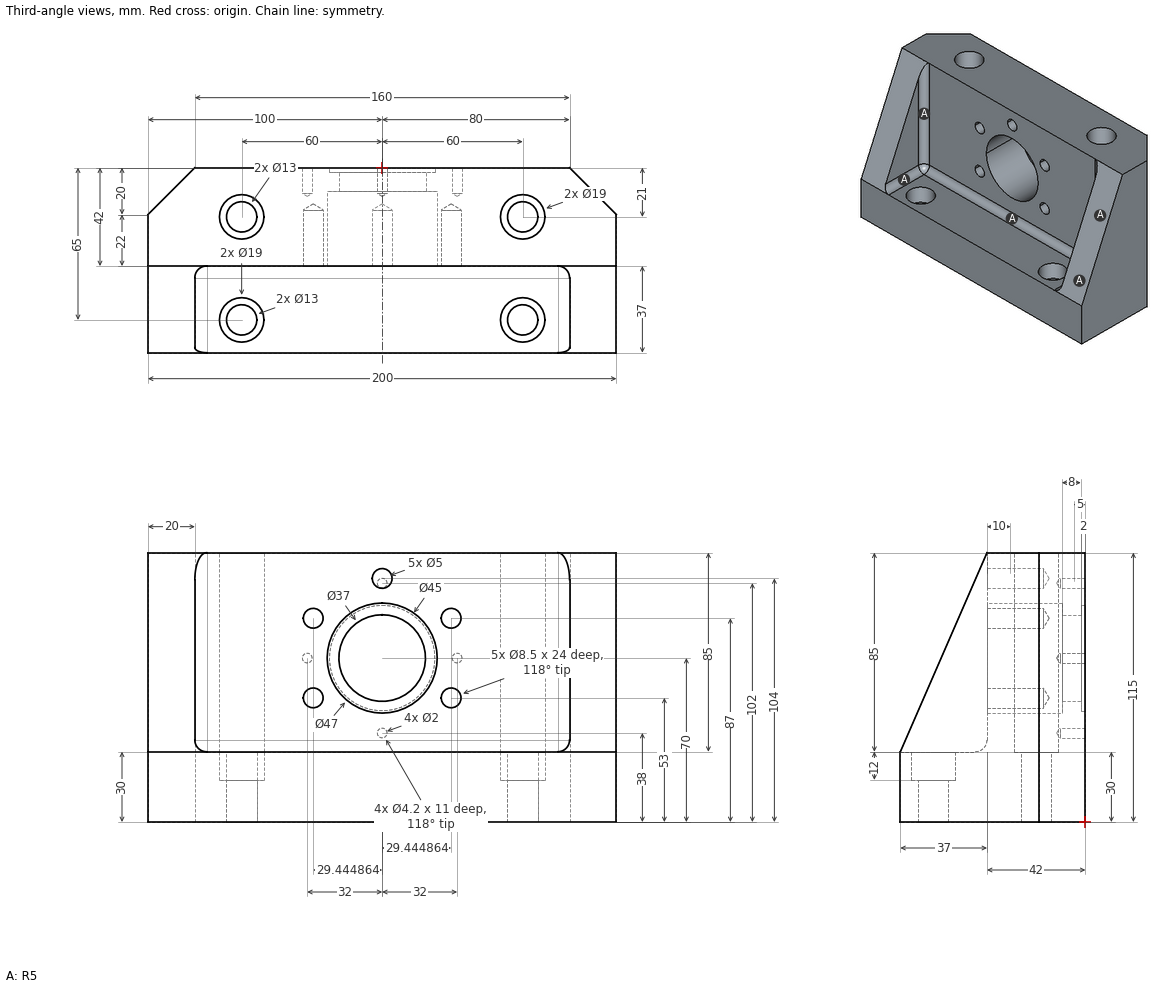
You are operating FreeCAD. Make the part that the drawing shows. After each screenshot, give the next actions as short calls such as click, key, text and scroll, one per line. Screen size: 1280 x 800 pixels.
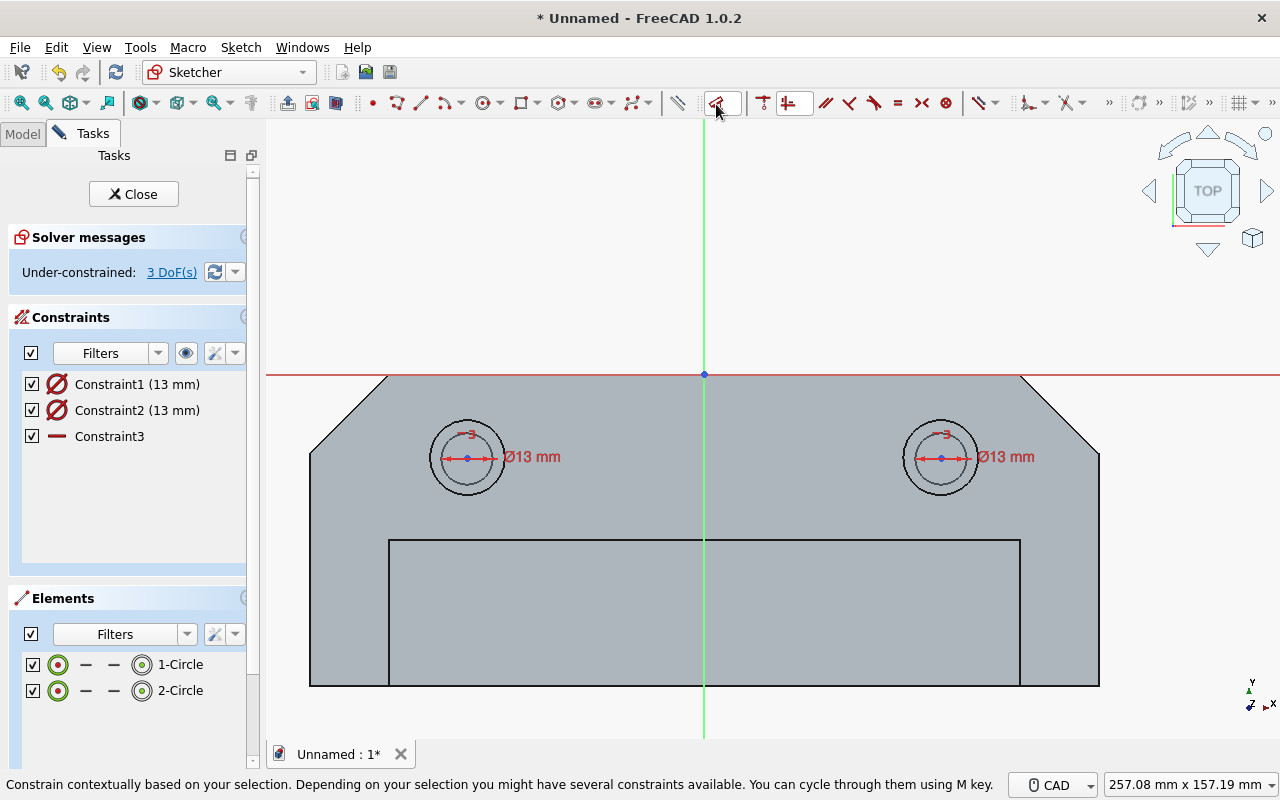
click(467, 459)
click(586, 341)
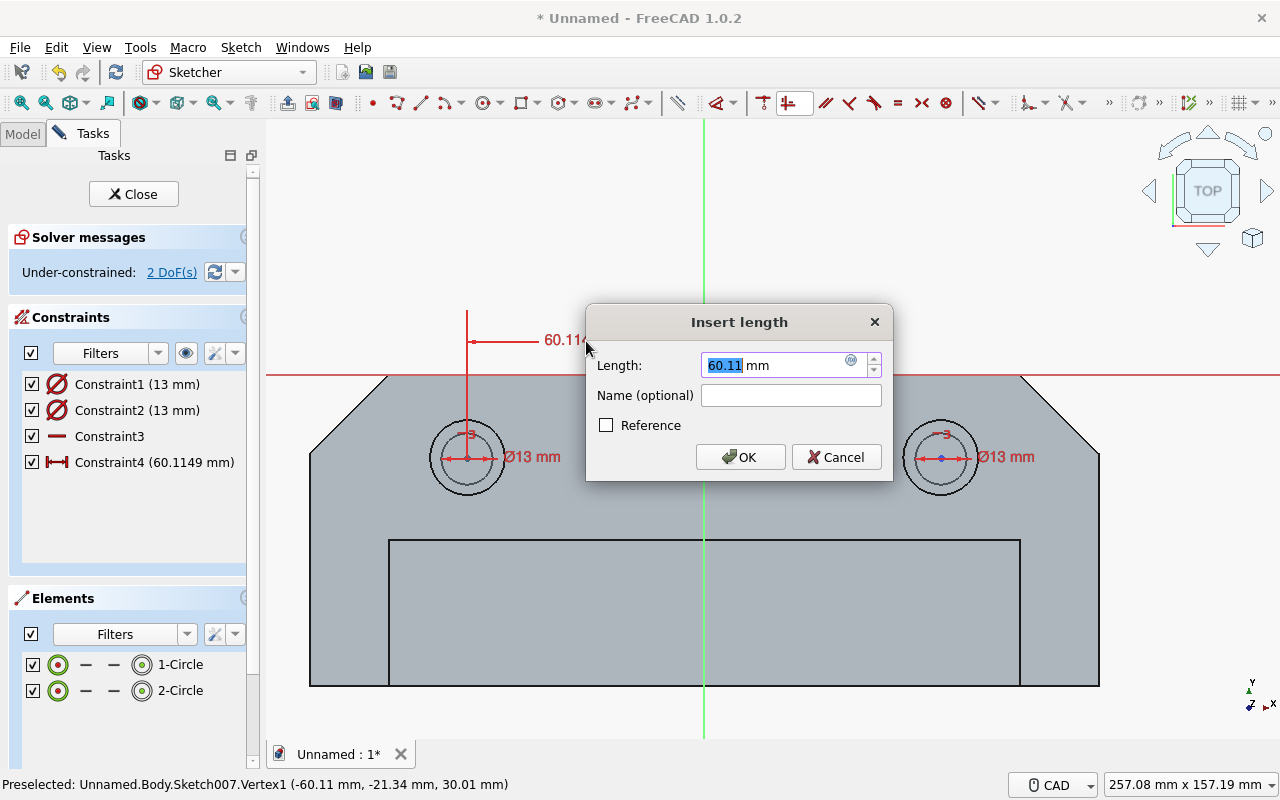
text(60)
key(Return)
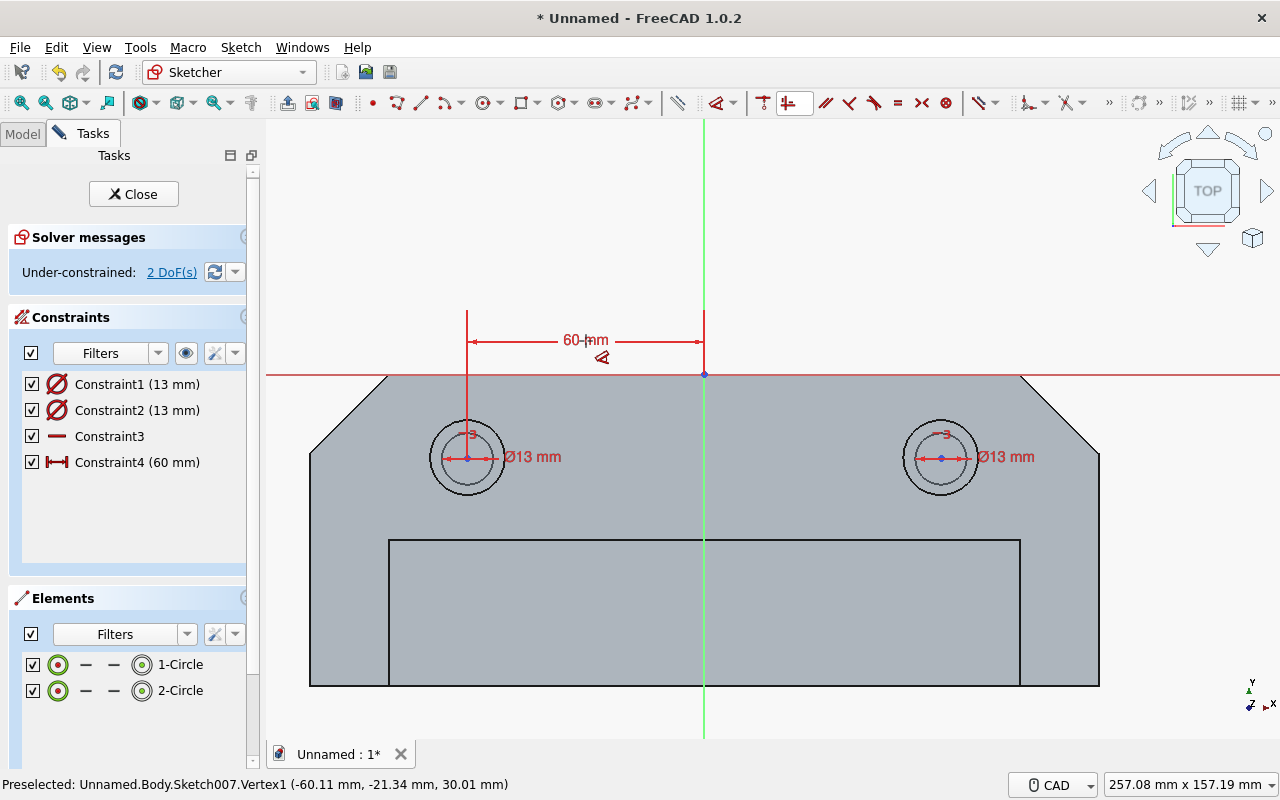
click(467, 459)
click(433, 417)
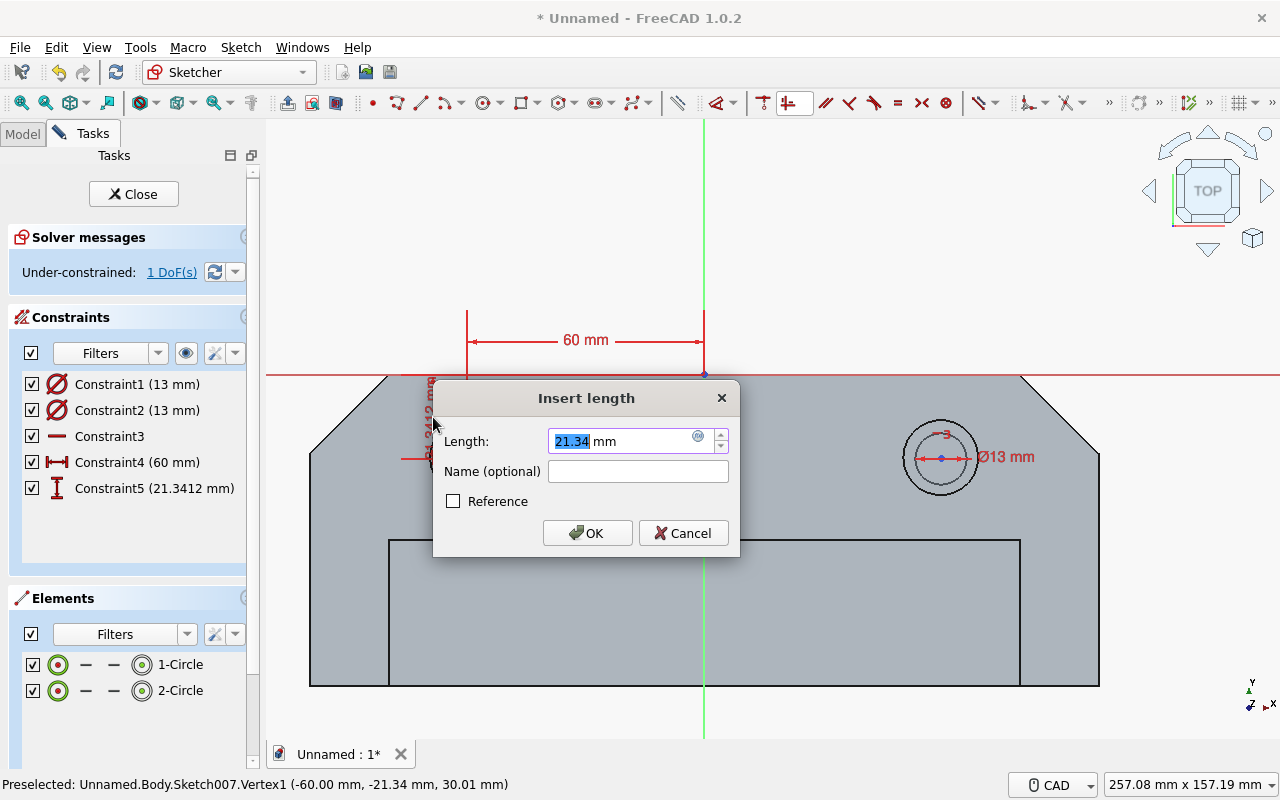
text(21)
key(Return)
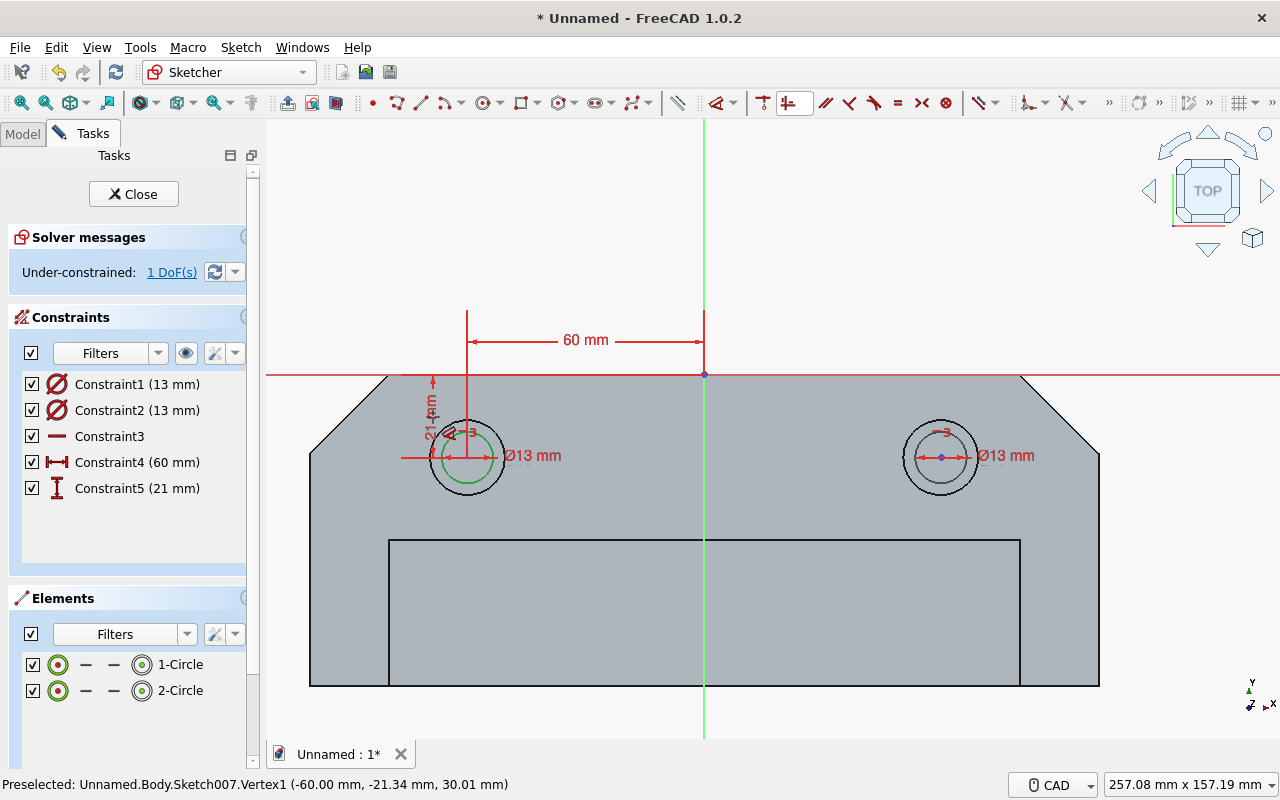
click(941, 458)
click(823, 341)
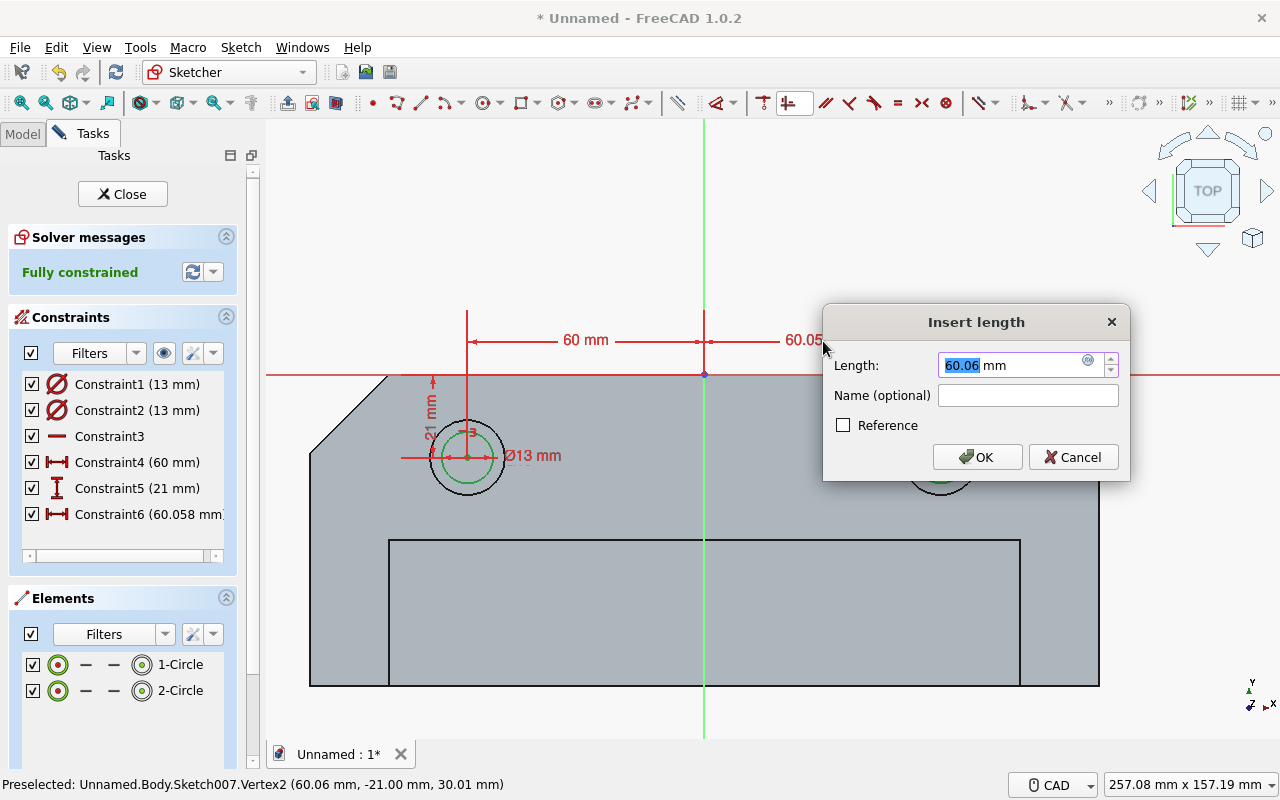
text(60)
key(Return)
key(Escape)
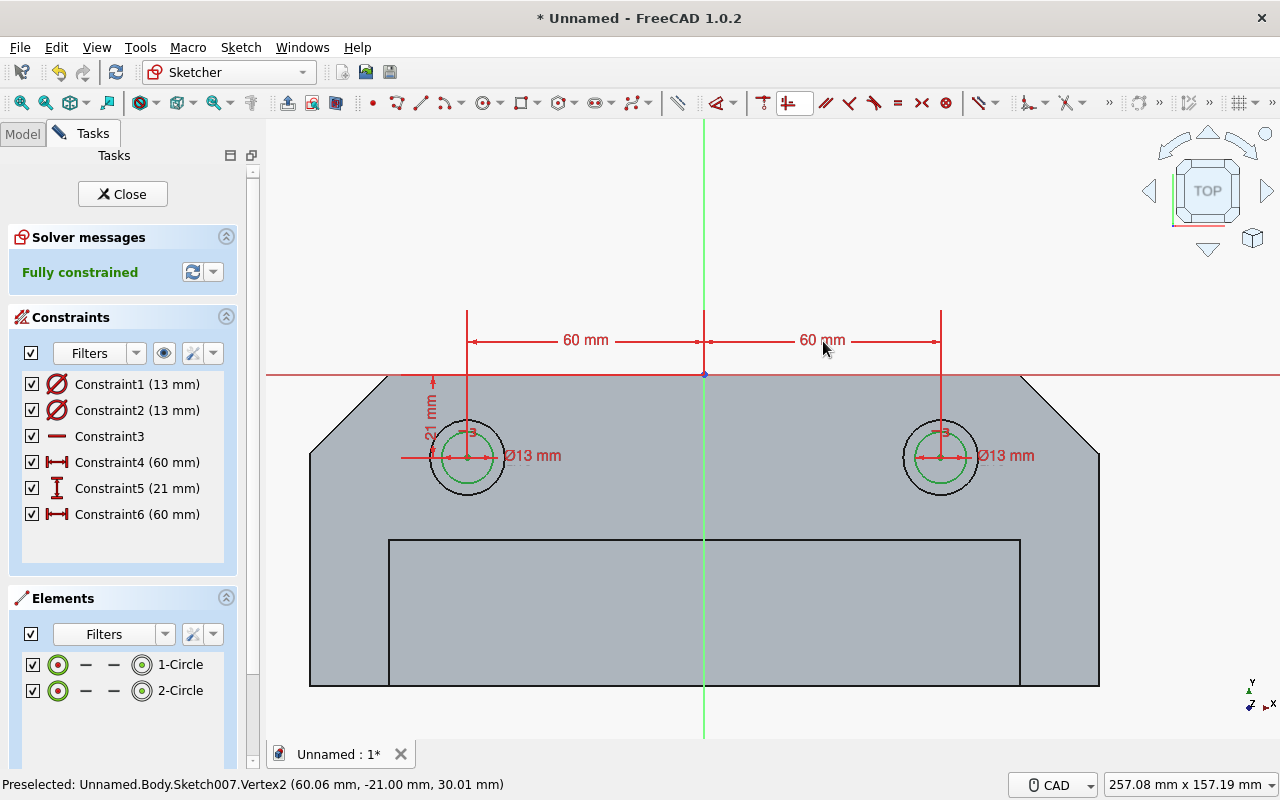
click(123, 194)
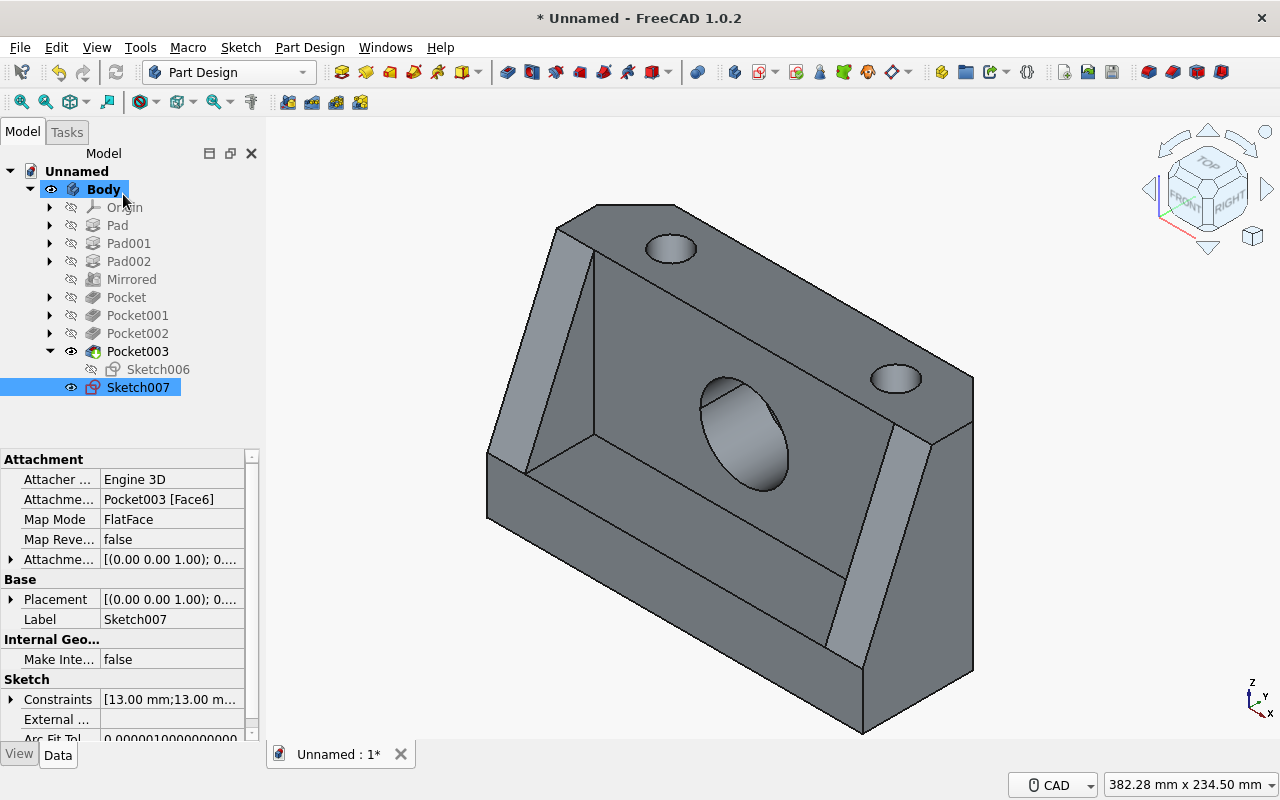
click(508, 72)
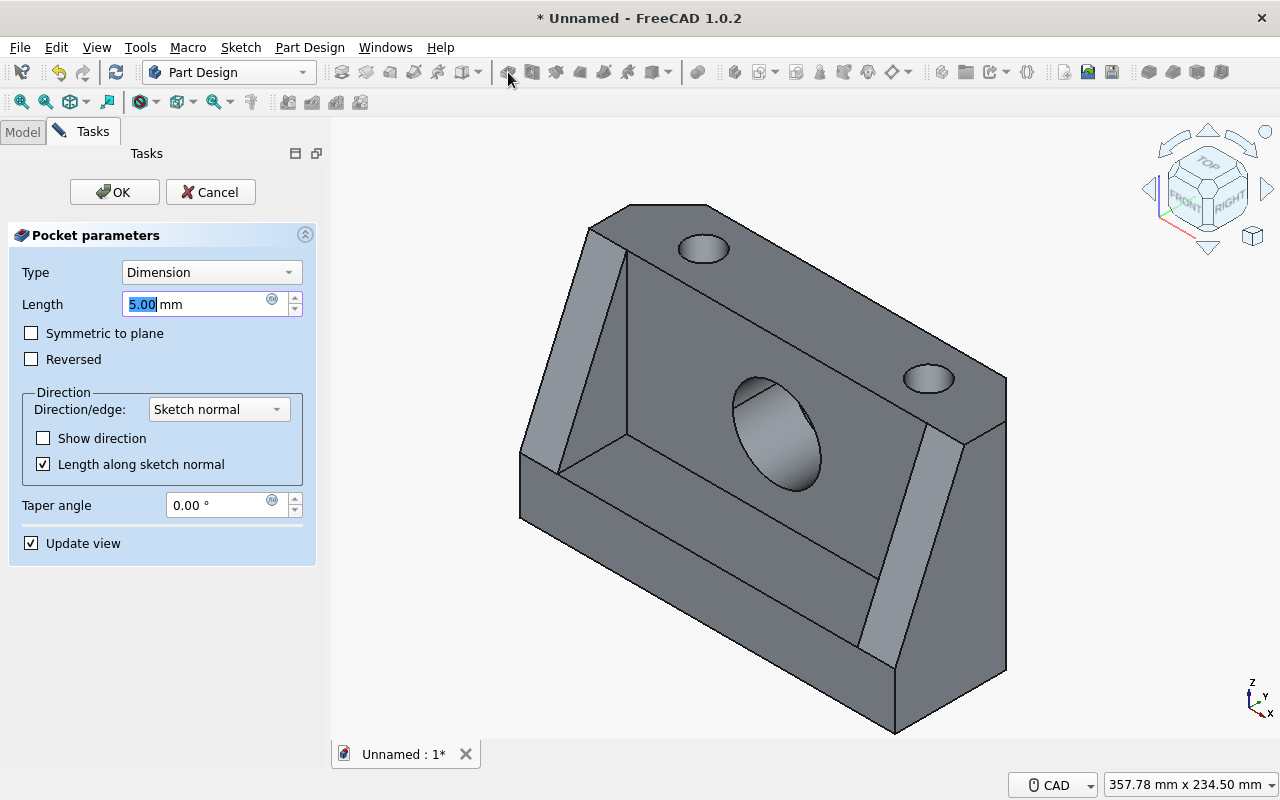
click(212, 272)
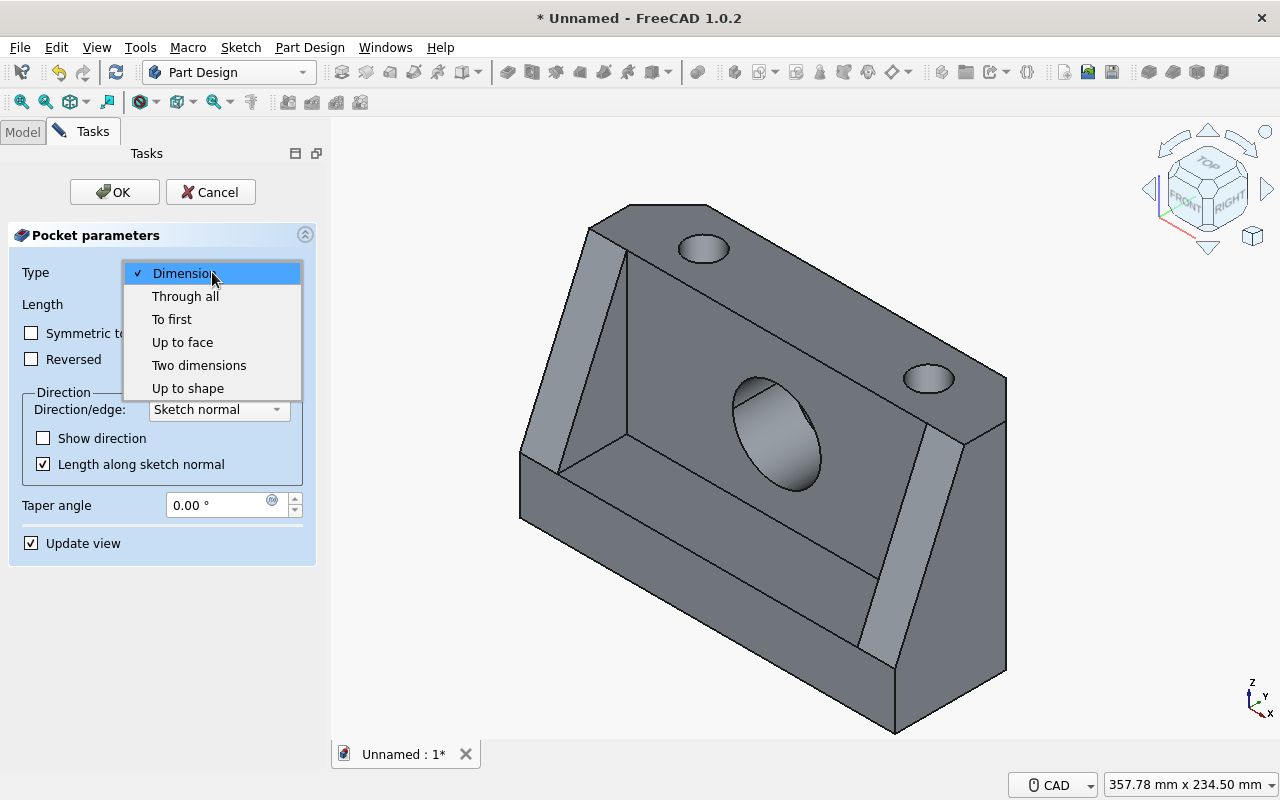
click(212, 296)